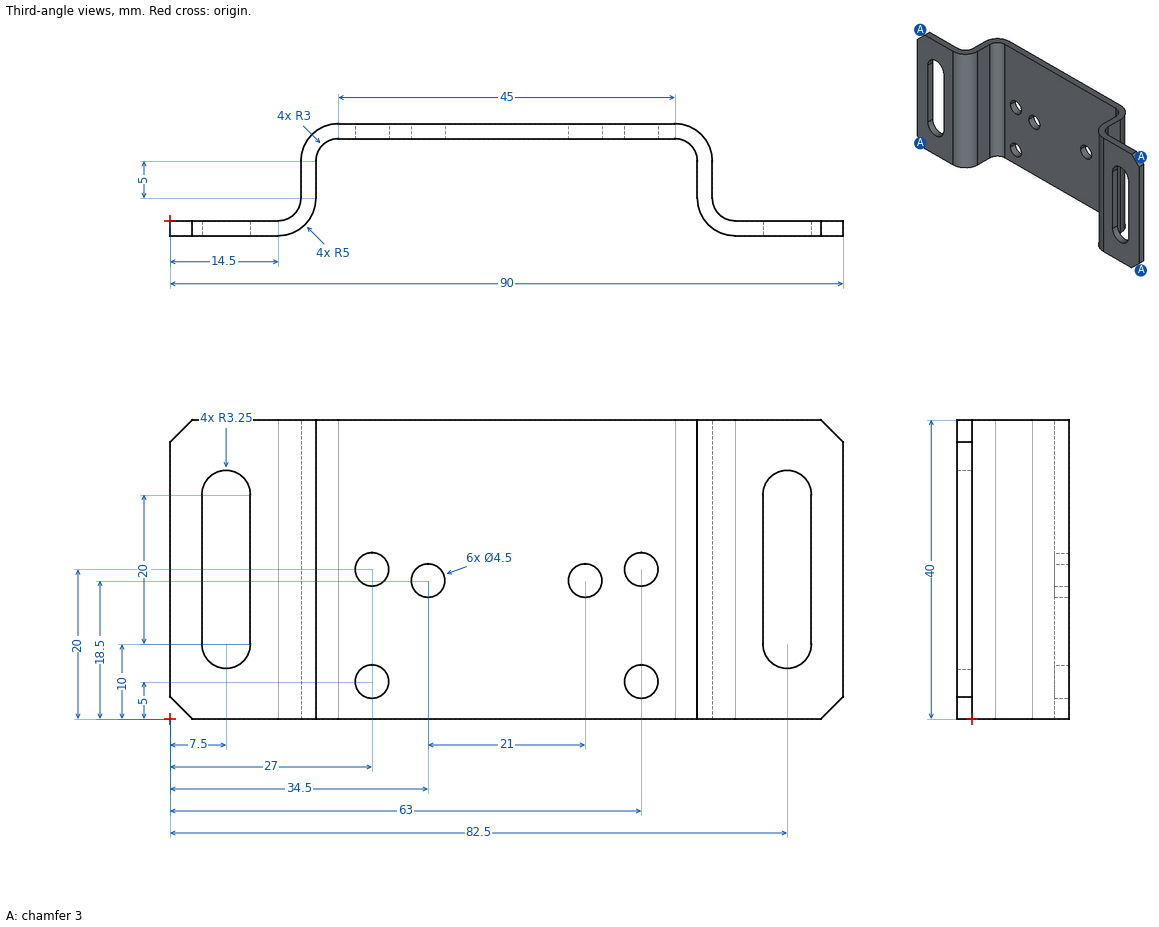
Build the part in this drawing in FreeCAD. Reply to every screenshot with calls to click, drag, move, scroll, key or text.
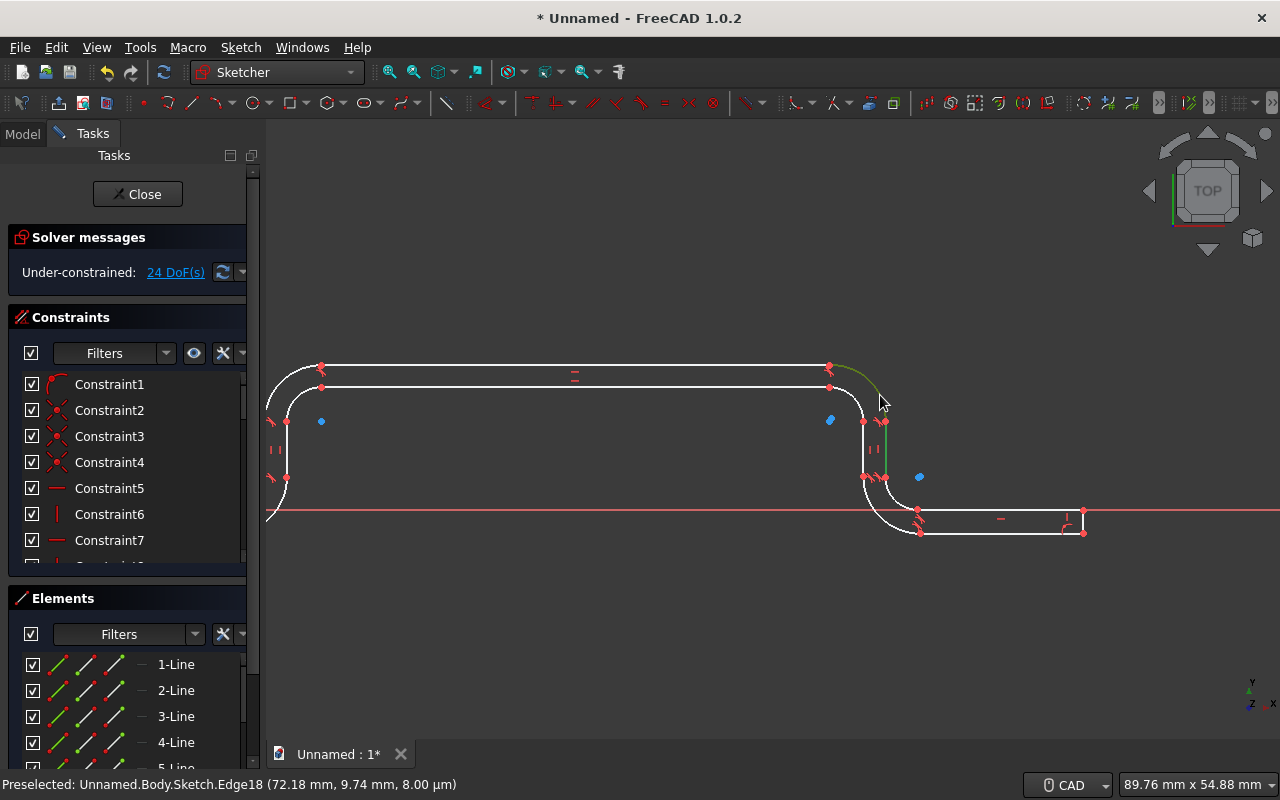
key(t)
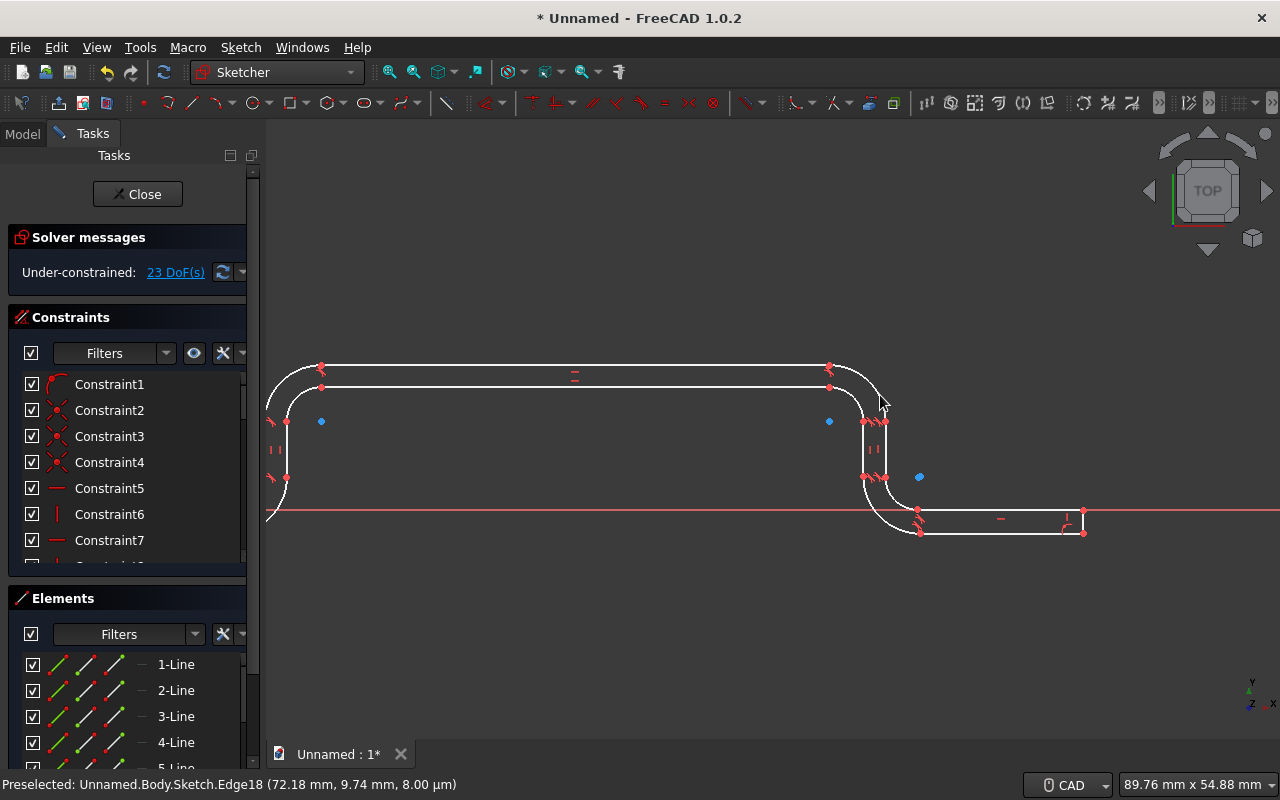
click(677, 365)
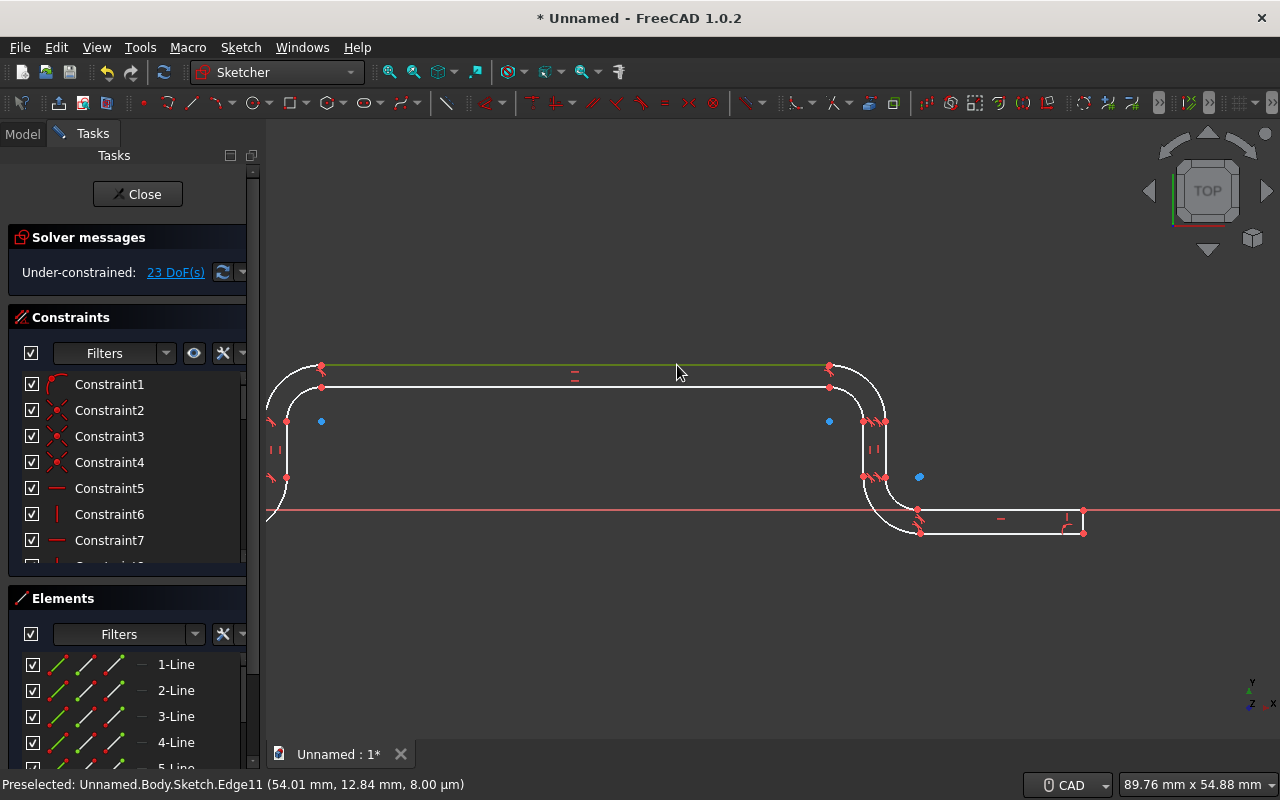
click(879, 396)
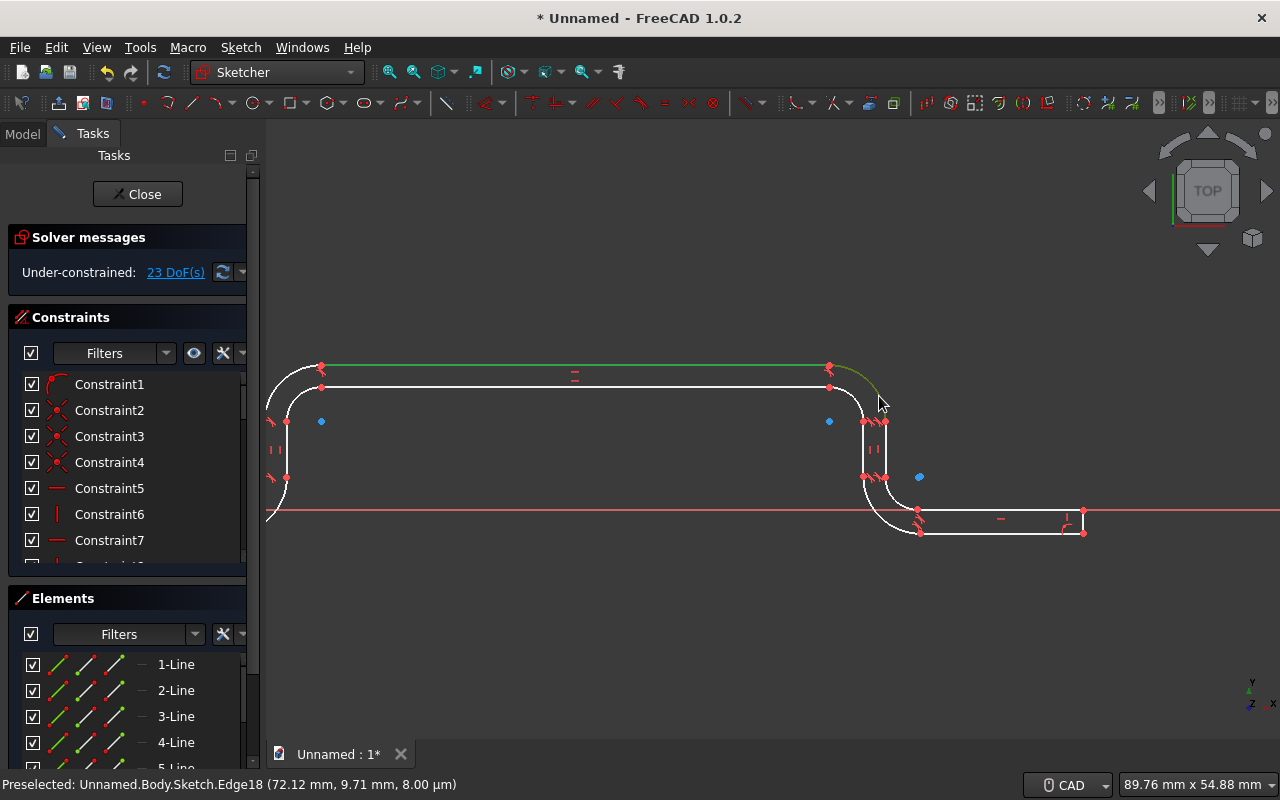
click(642, 104)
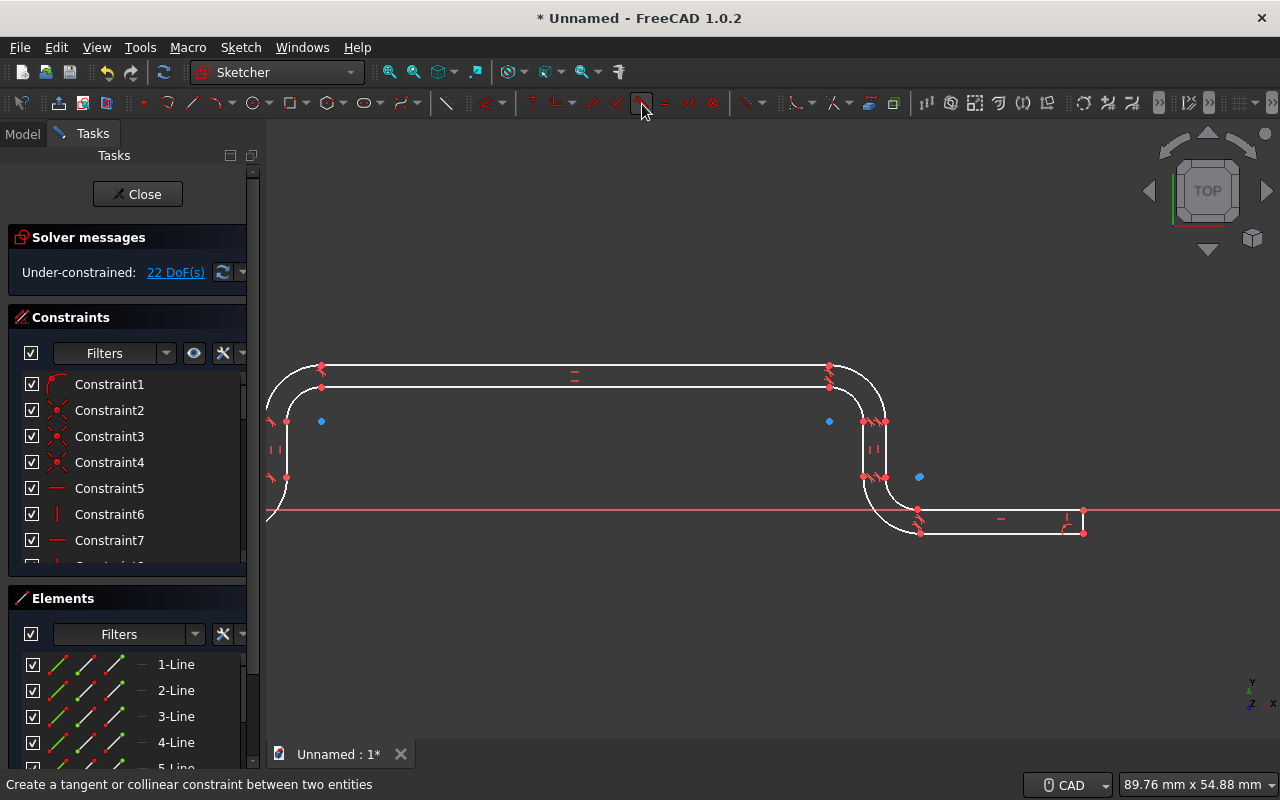
click(677, 365)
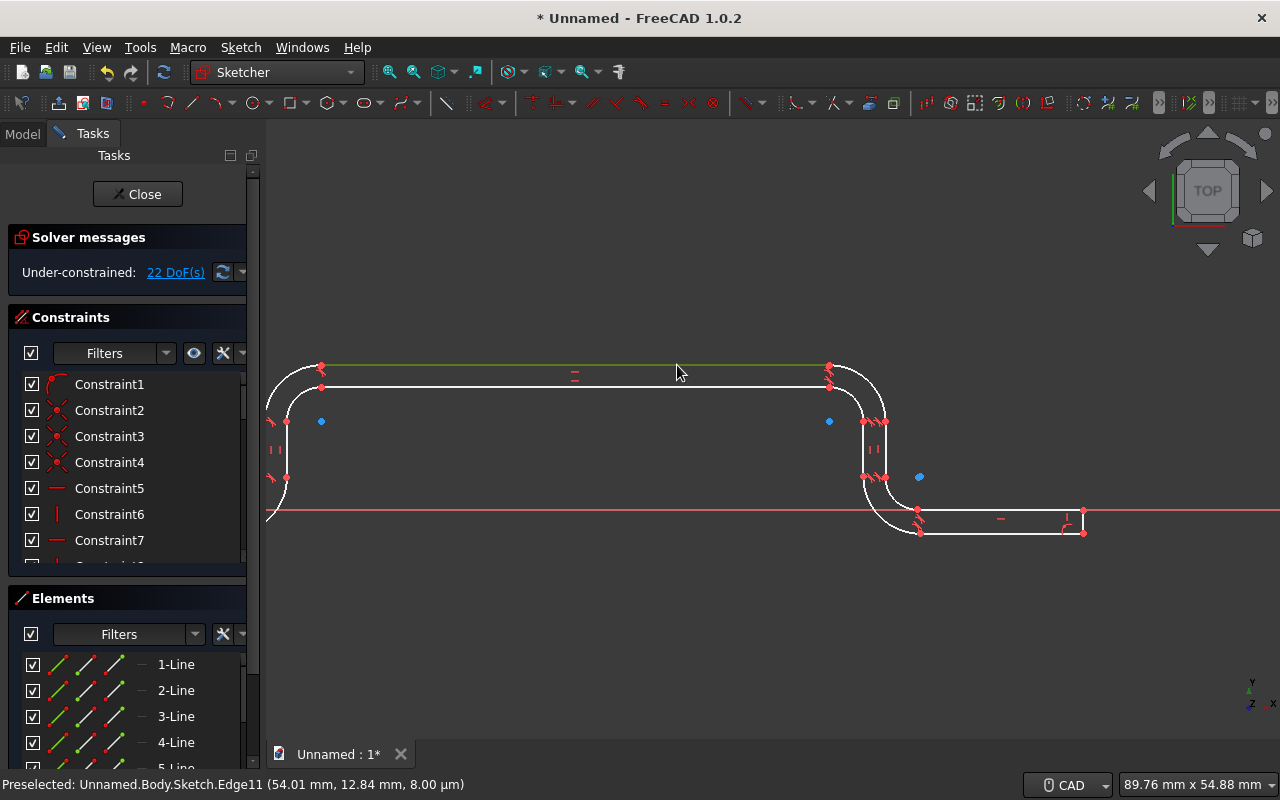
click(296, 371)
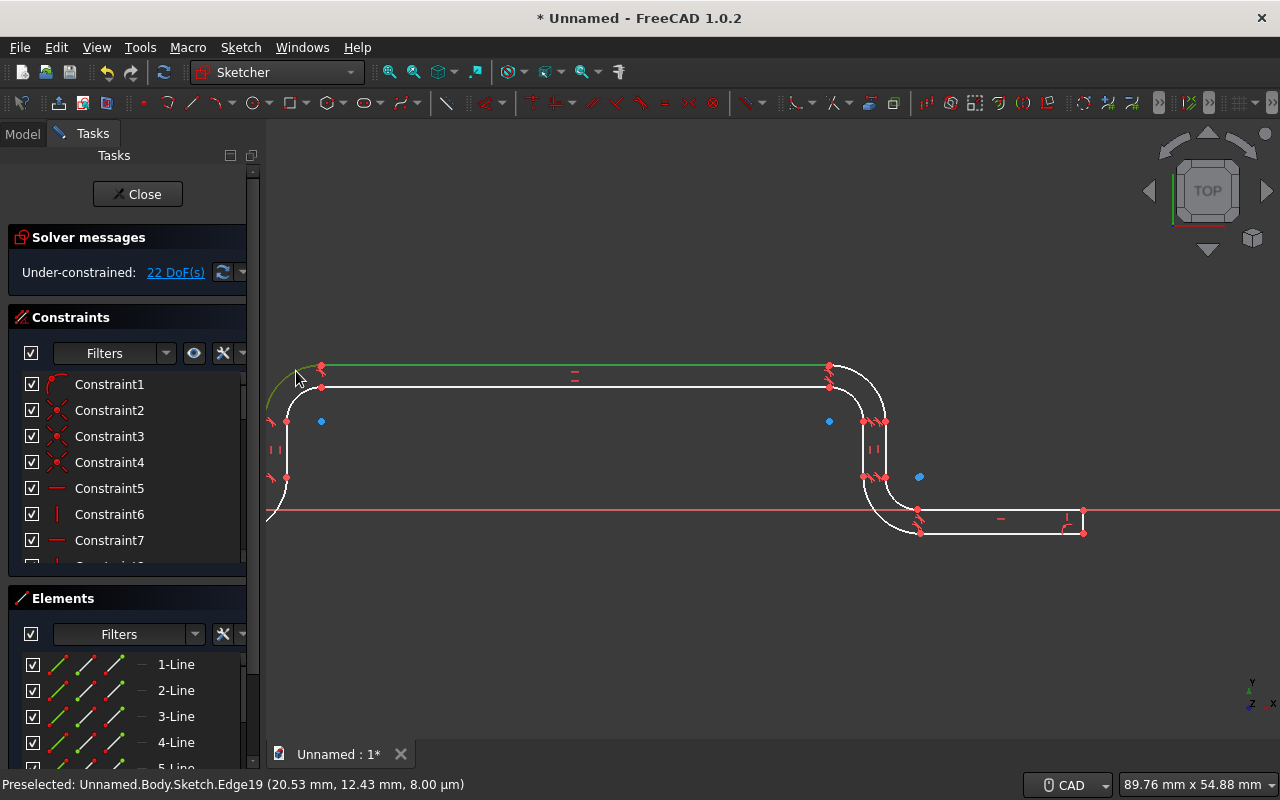
key(t)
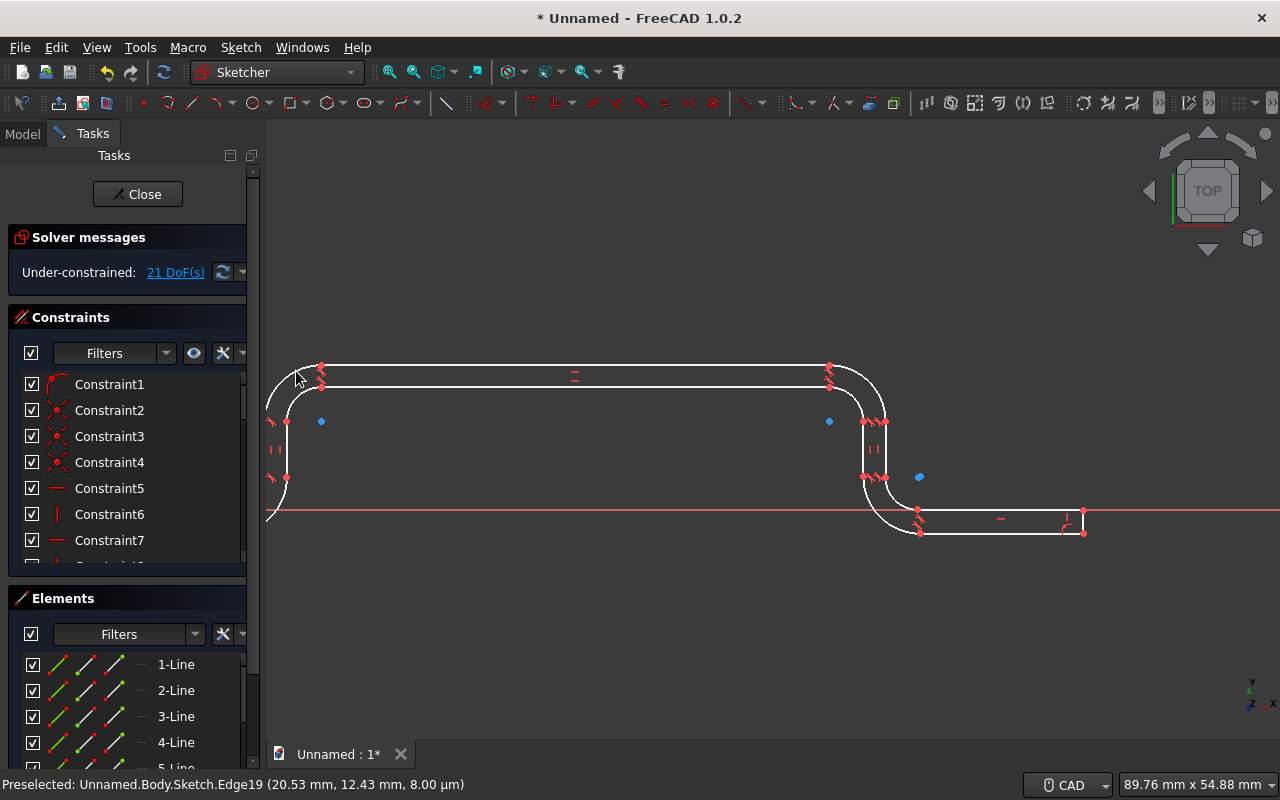
scroll(862, 406, down, 3)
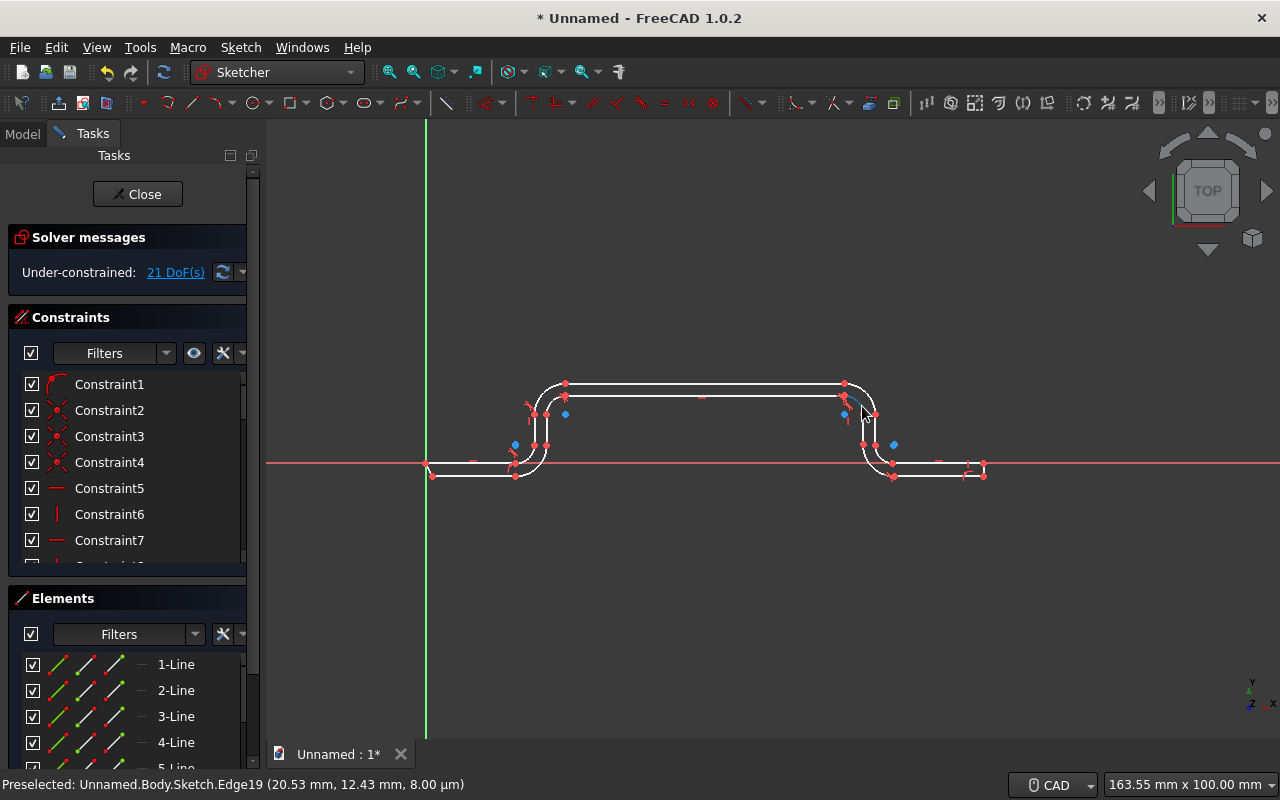
scroll(535, 424, up, 3)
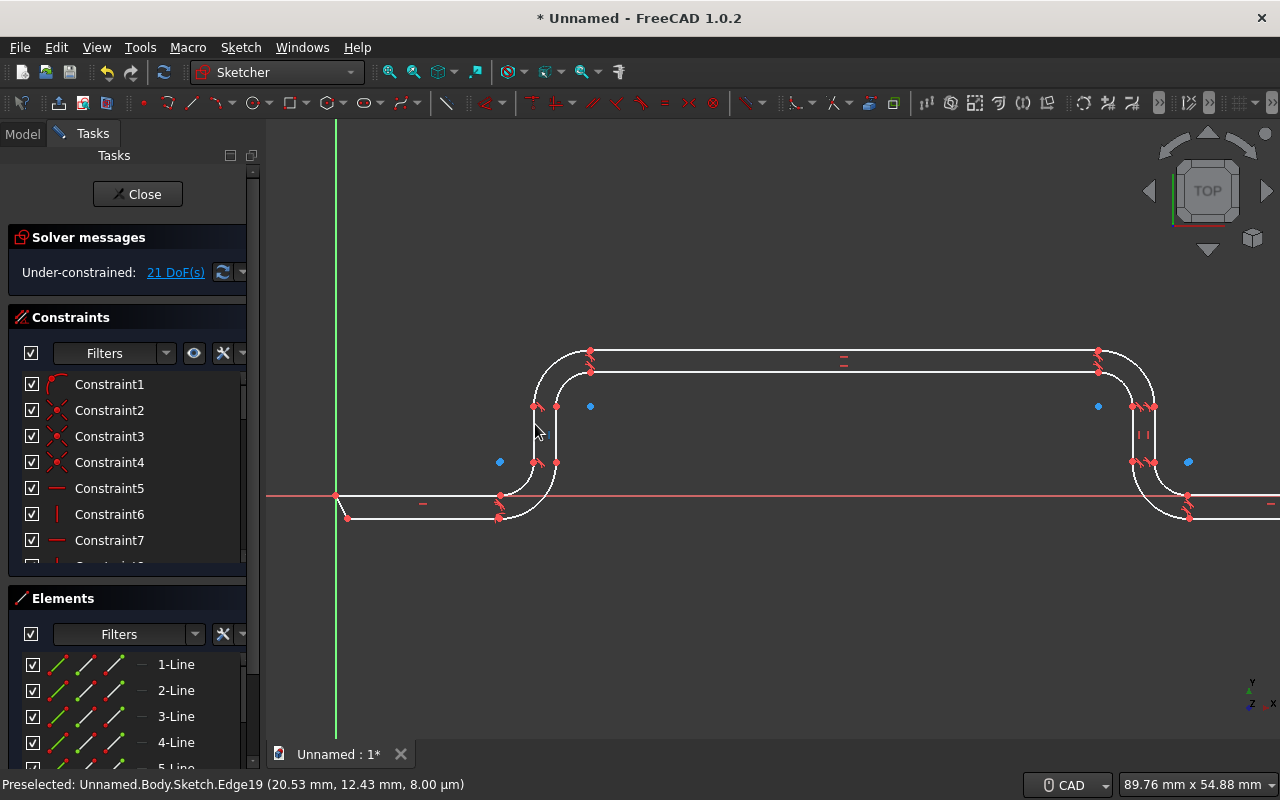
click(534, 423)